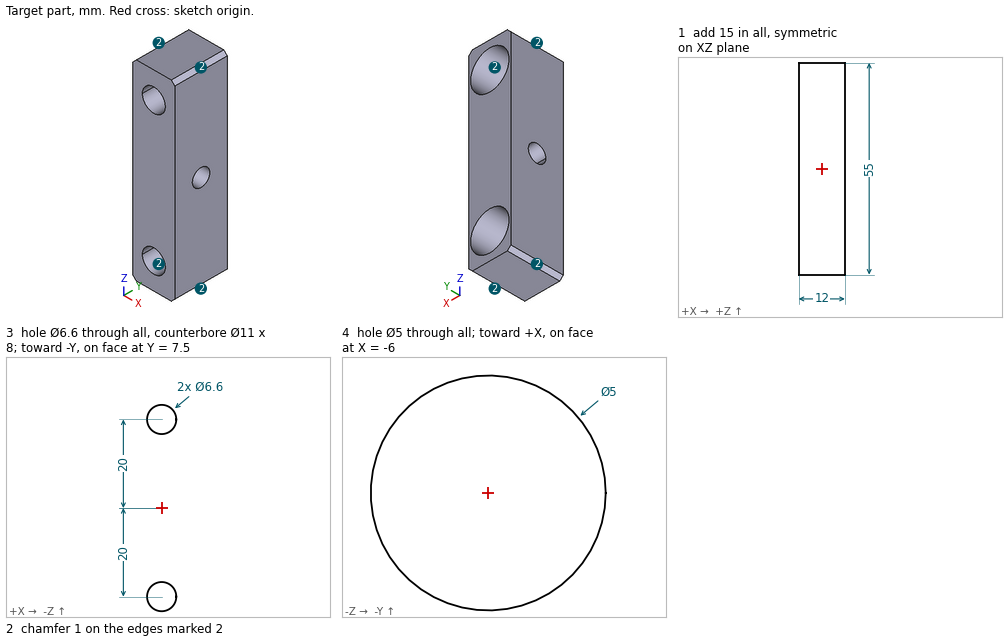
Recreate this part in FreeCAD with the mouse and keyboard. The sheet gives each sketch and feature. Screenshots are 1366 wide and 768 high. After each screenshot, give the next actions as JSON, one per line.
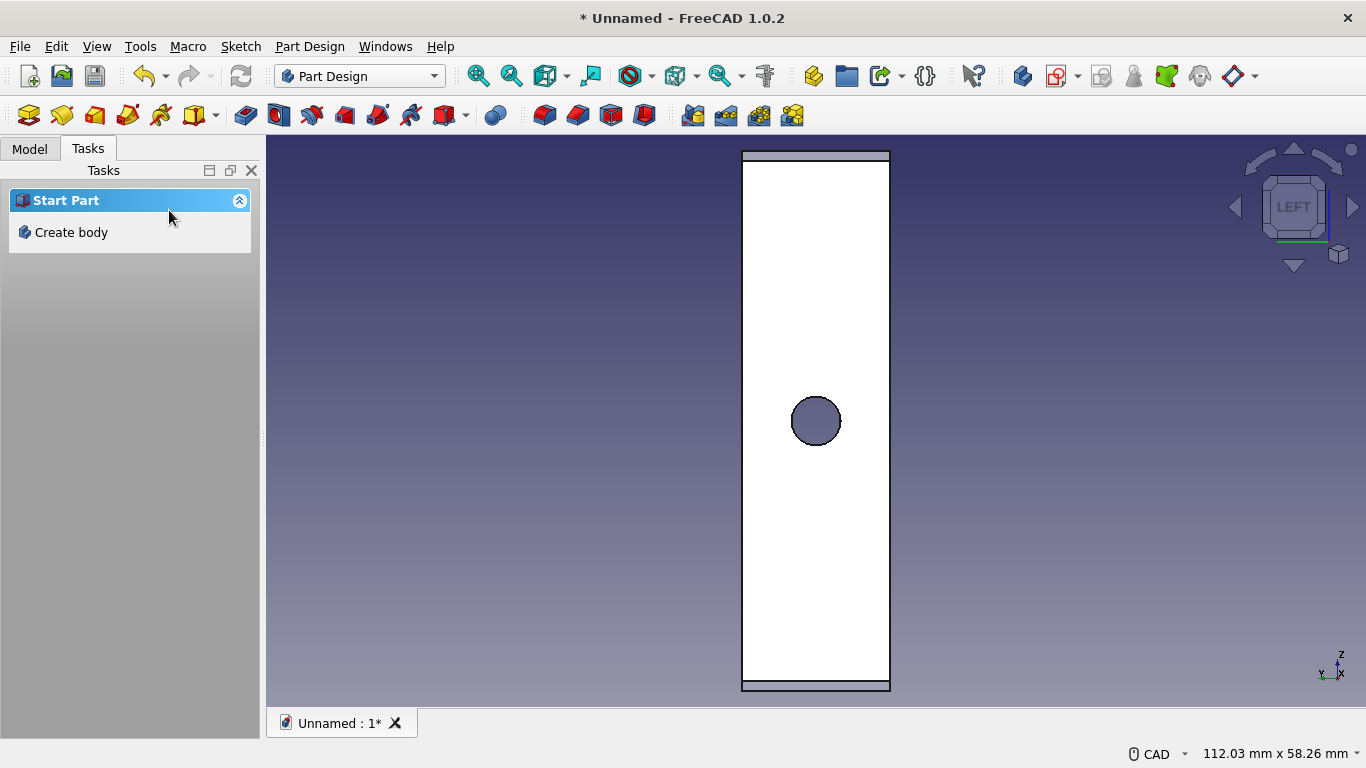
{"action": "key", "text": "0"}